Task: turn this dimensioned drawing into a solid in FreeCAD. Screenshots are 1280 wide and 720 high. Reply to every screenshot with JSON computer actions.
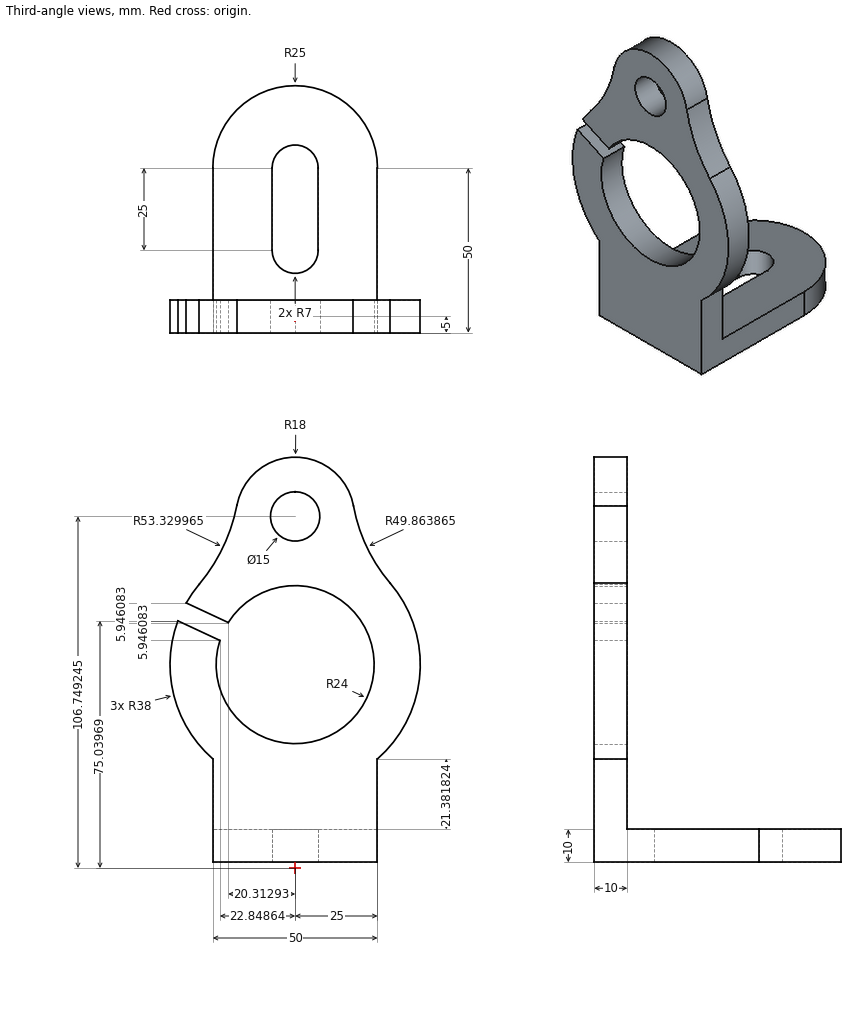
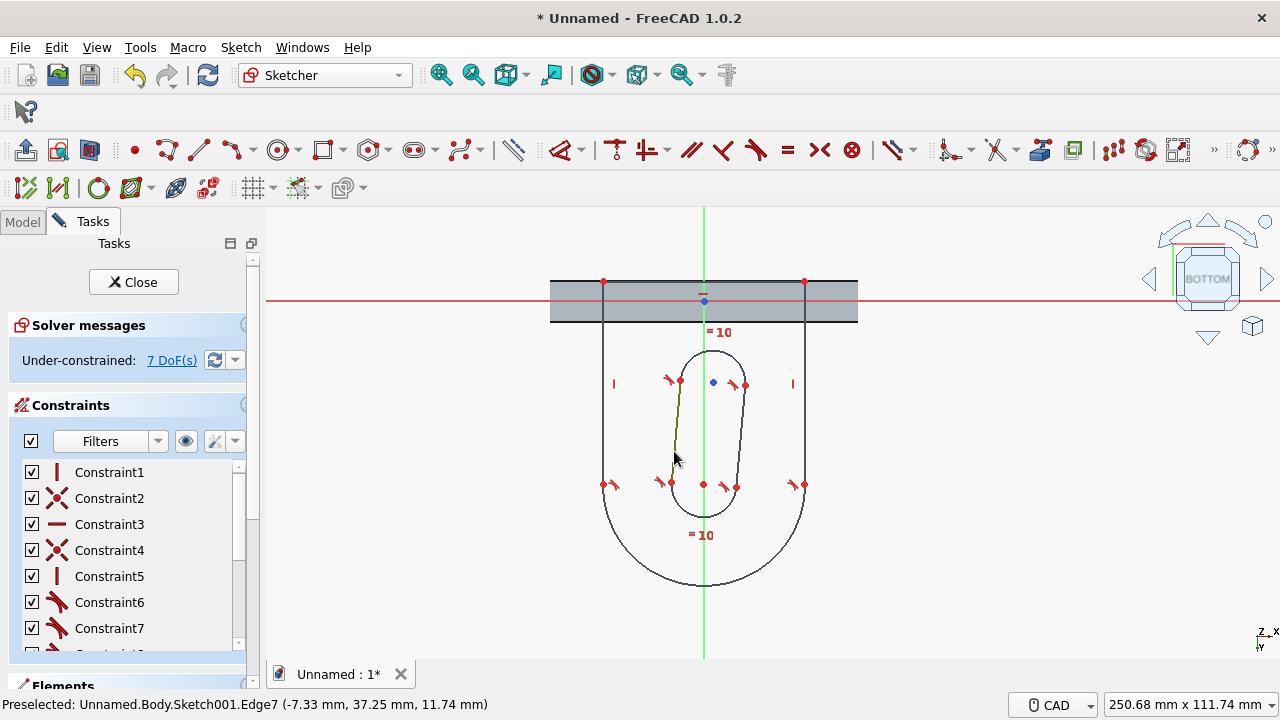
{"action": "key", "text": "v"}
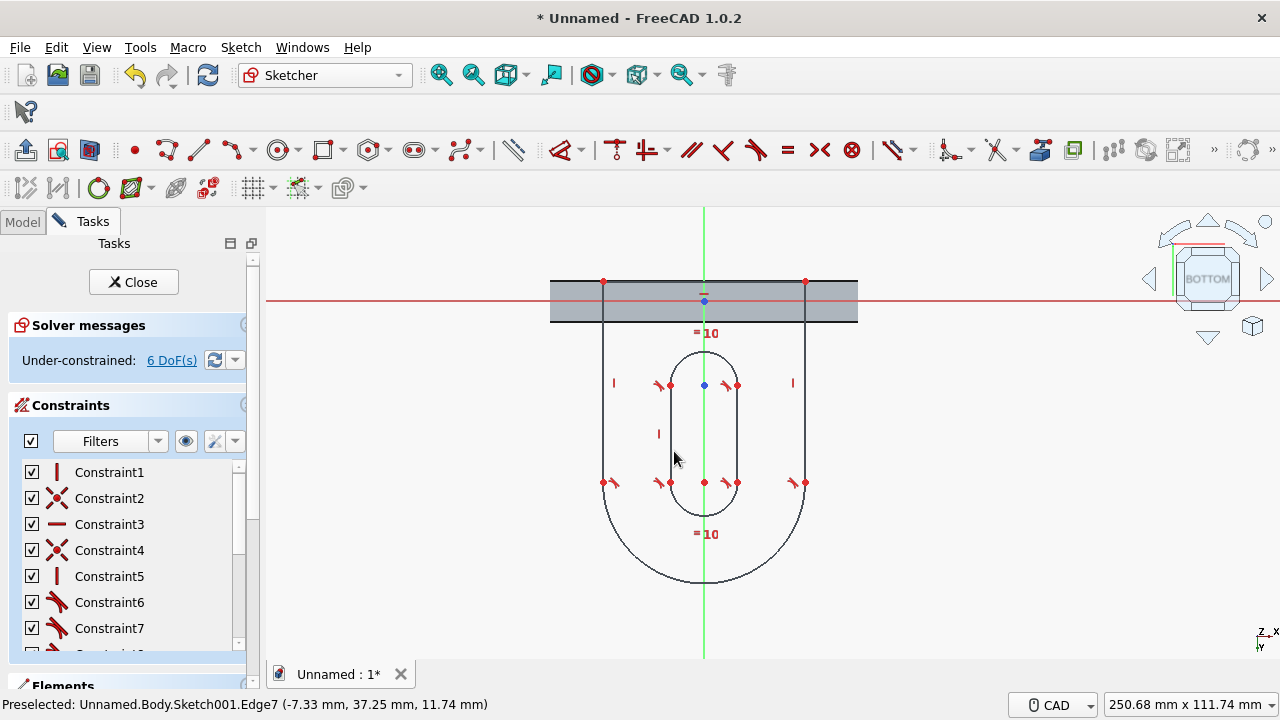
{"action": "left_click", "coordinate": [704, 482]}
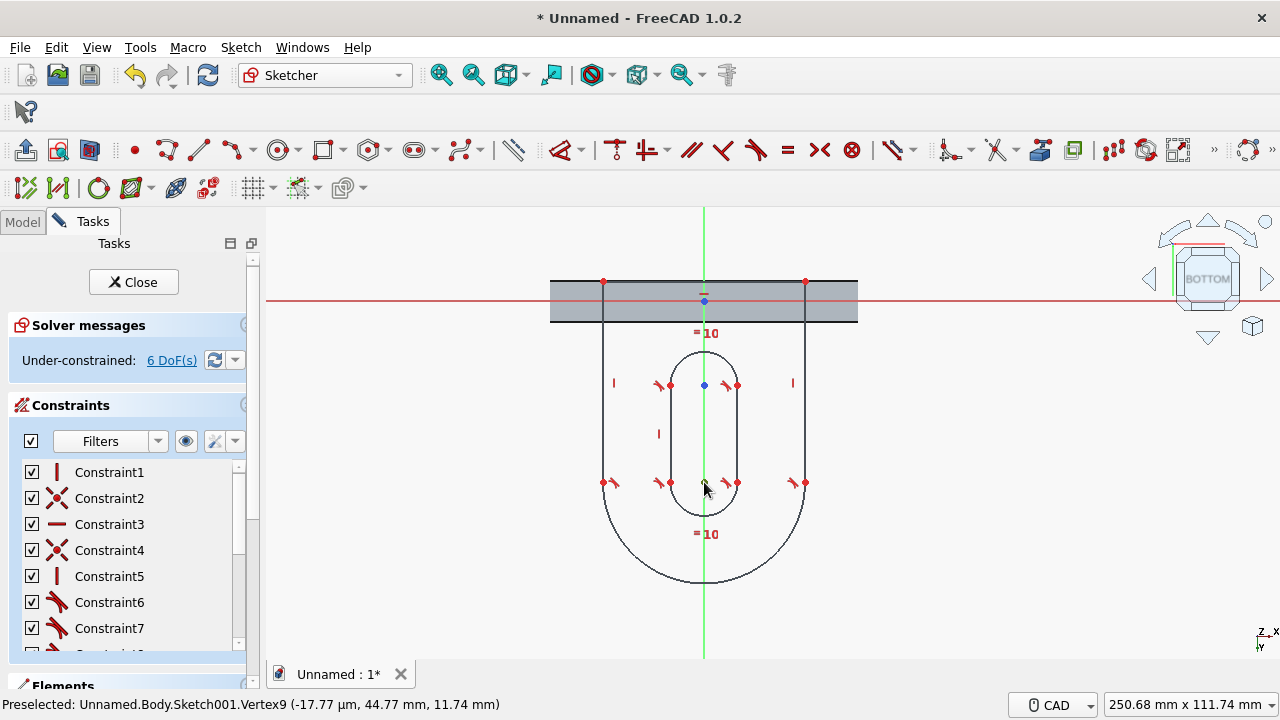
{"action": "left_click", "coordinate": [704, 546]}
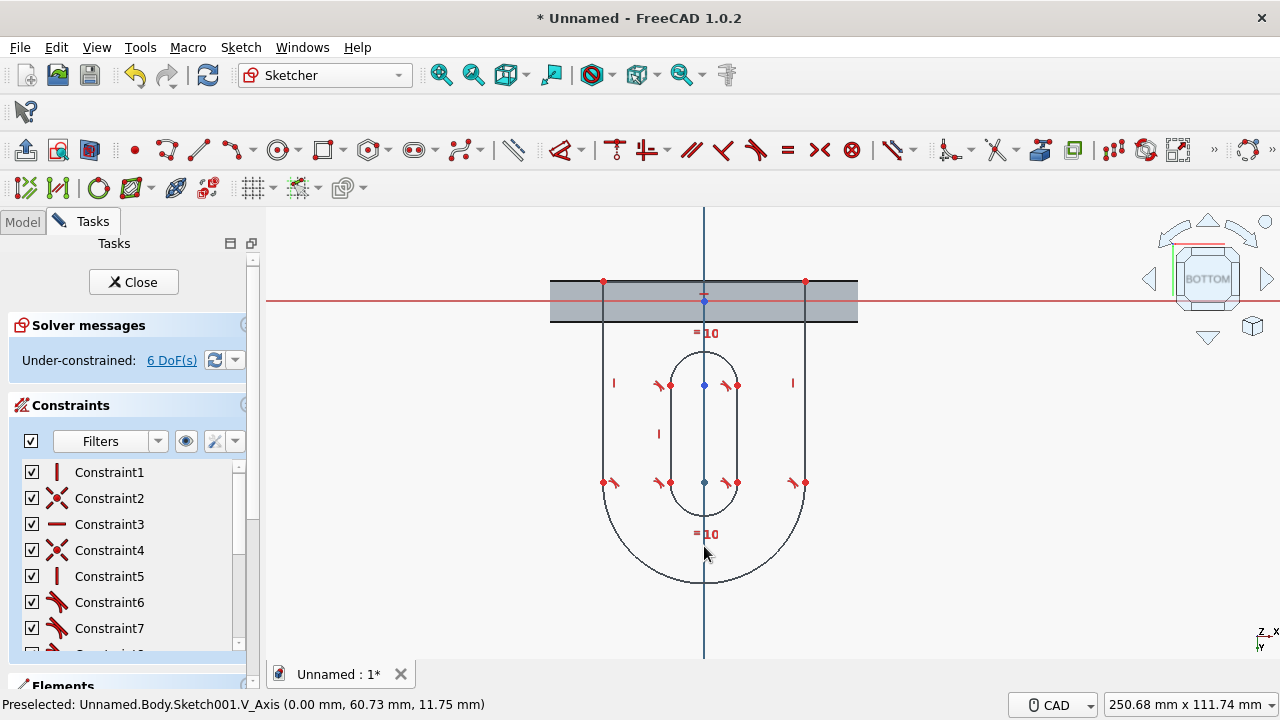
{"action": "left_click", "coordinate": [616, 150]}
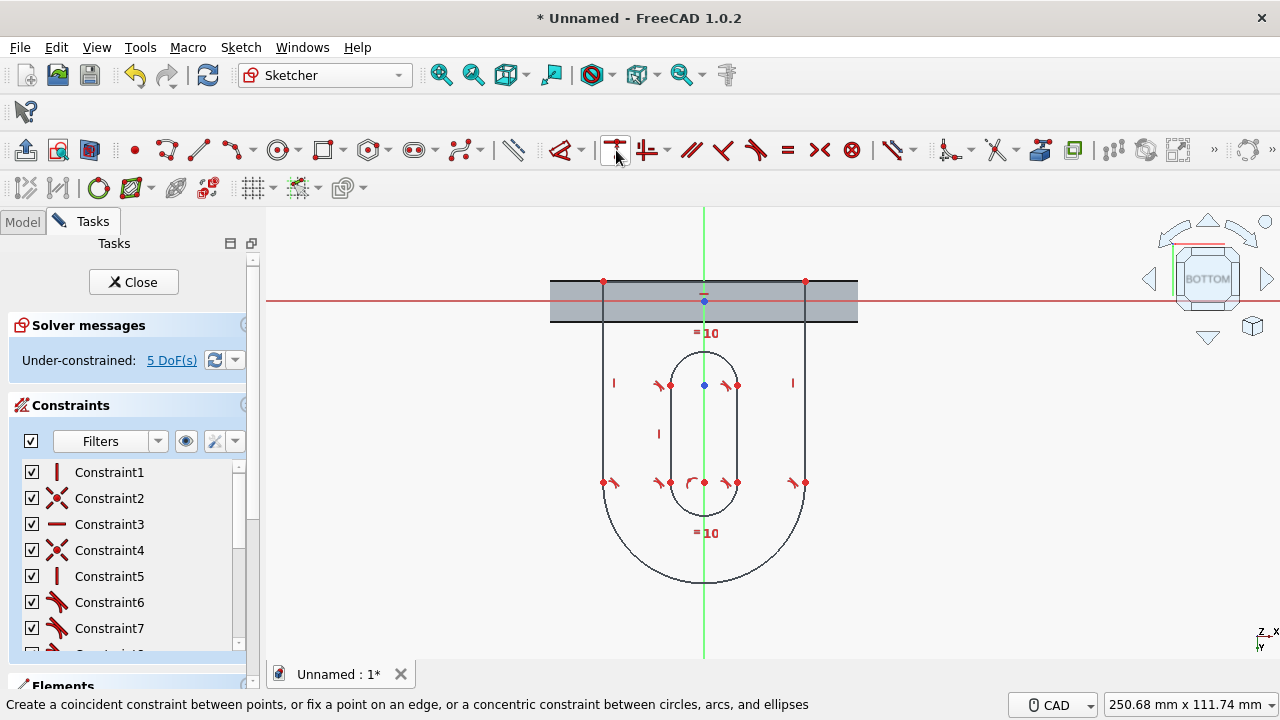
{"action": "left_click", "coordinate": [560, 150]}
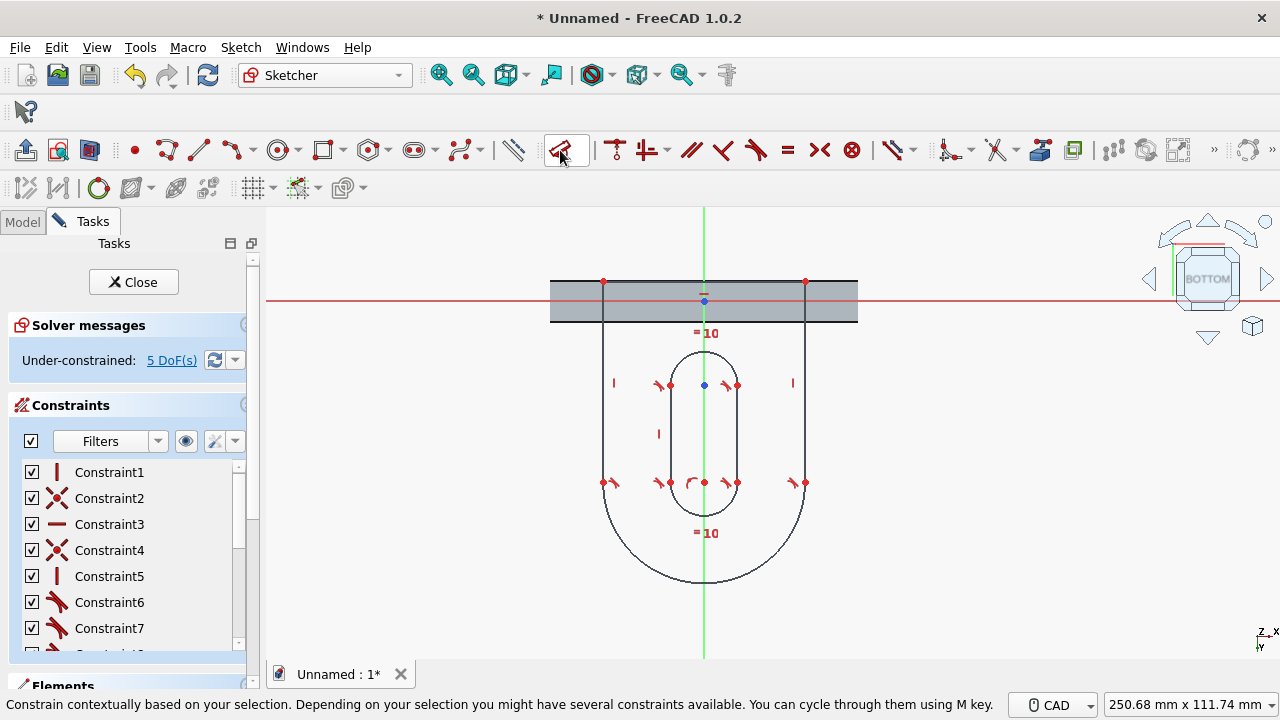
{"action": "left_click", "coordinate": [645, 564]}
{"action": "left_click", "coordinate": [626, 590]}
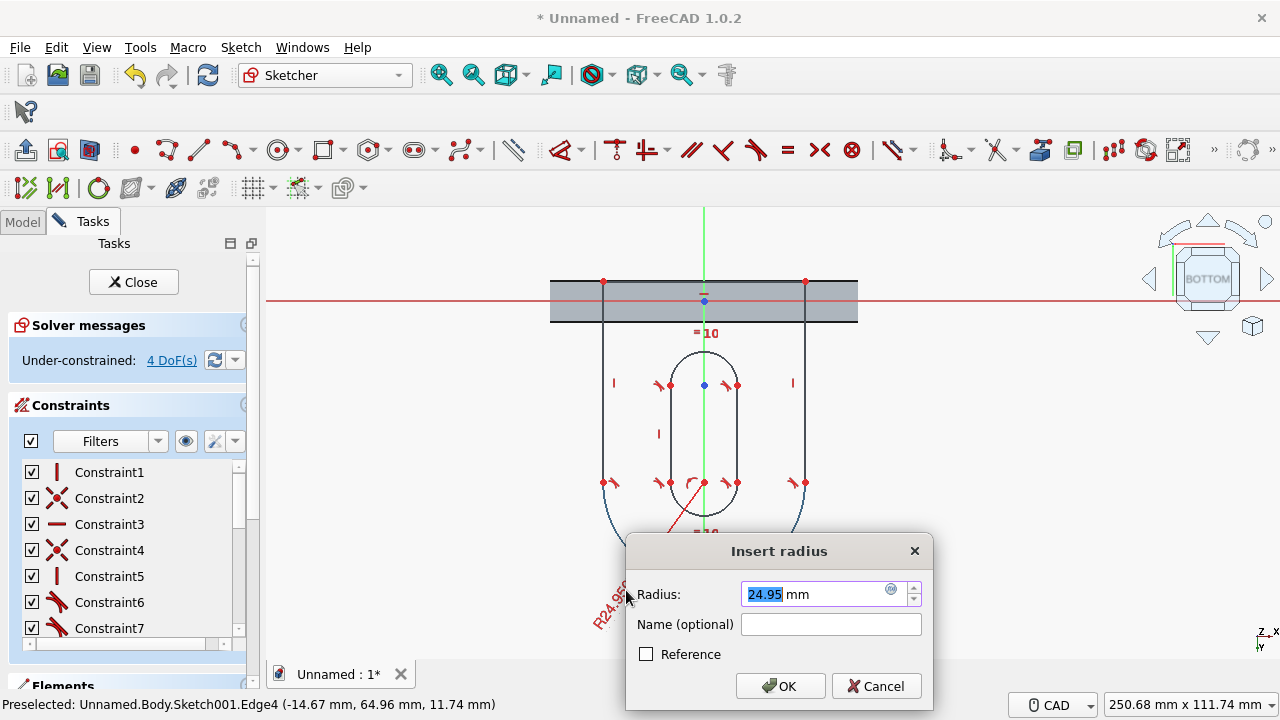
{"action": "type", "text": "25"}
{"action": "key", "text": "Return"}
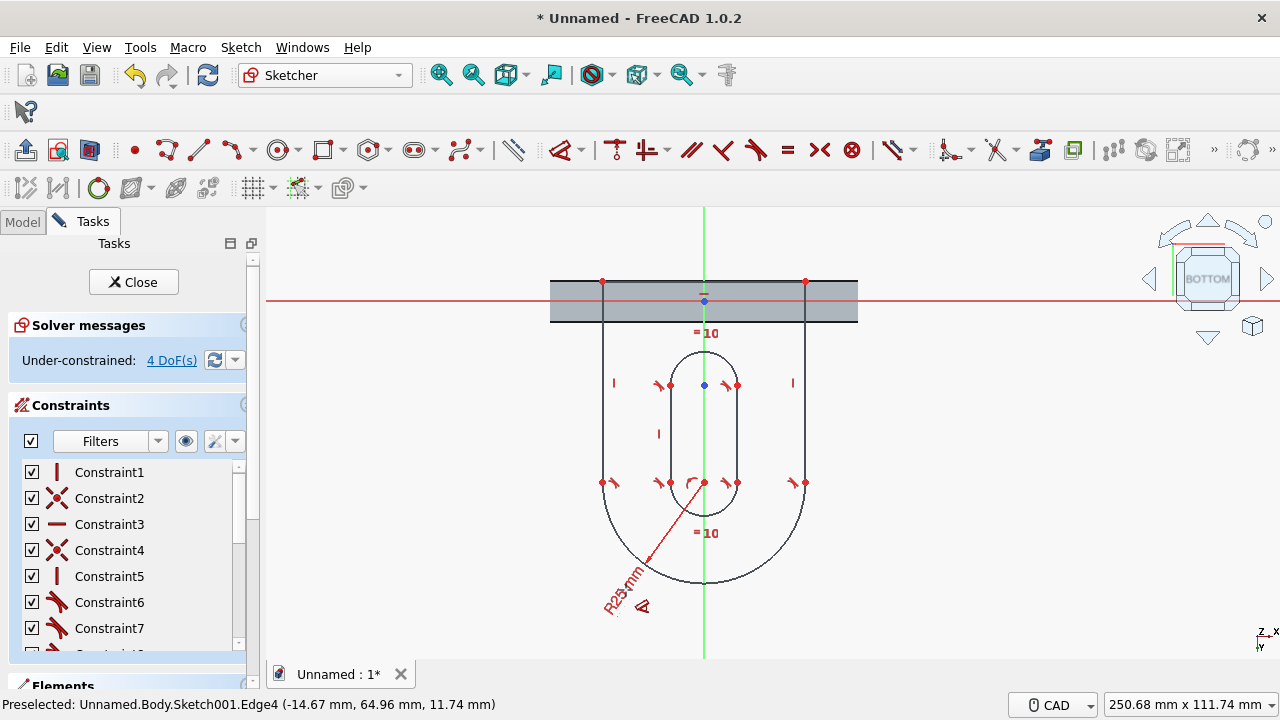
{"action": "scroll", "coordinate": [684, 509], "scroll_direction": "up", "scroll_amount": 2}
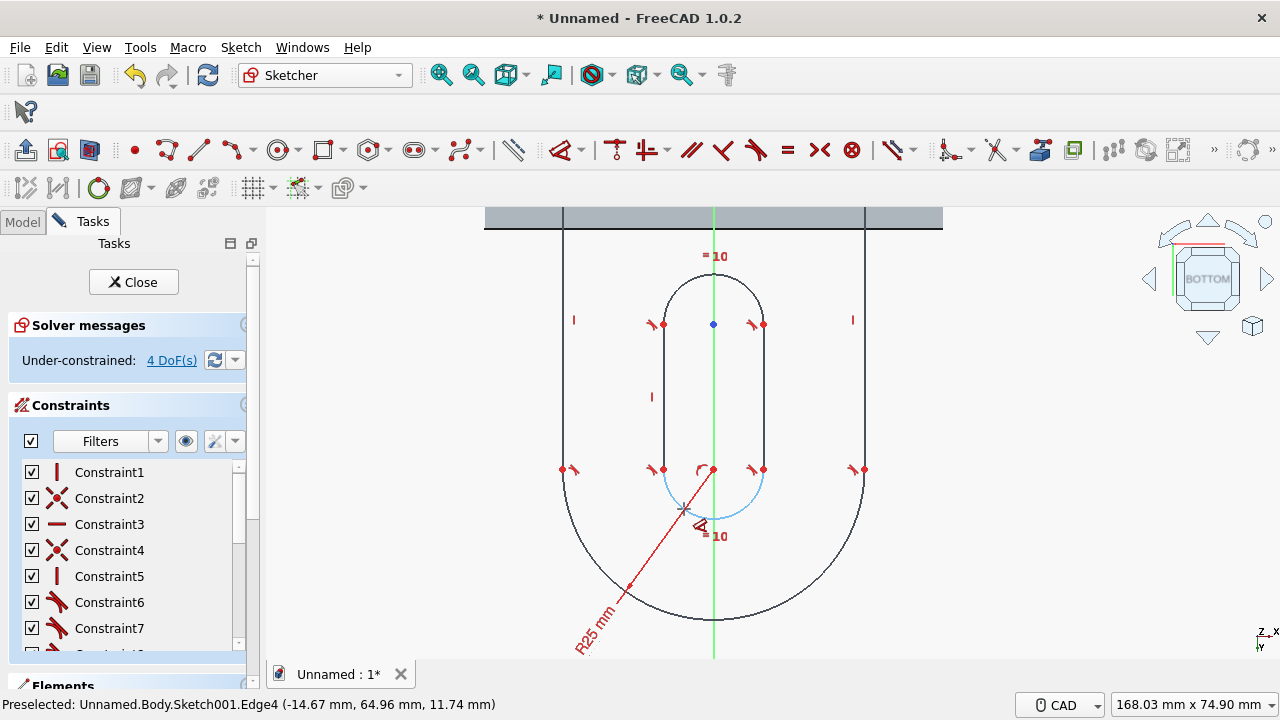
{"action": "left_click", "coordinate": [684, 509]}
{"action": "left_click", "coordinate": [665, 535]}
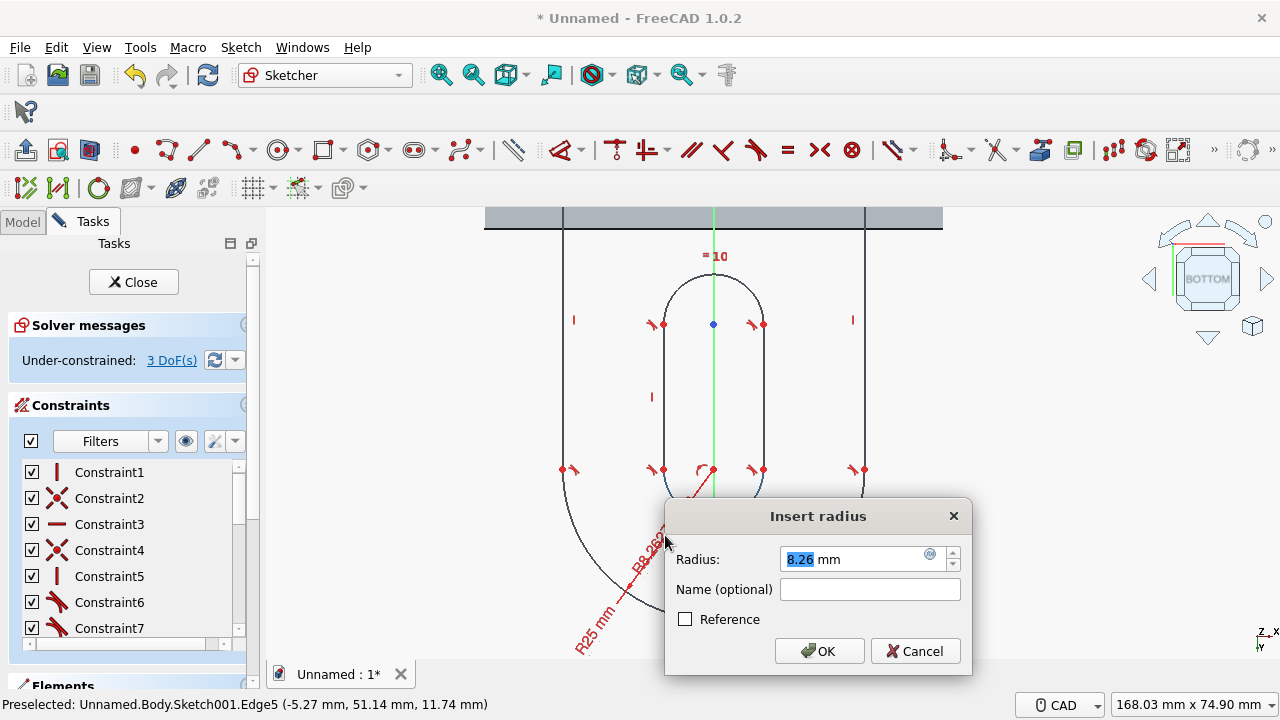
{"action": "type", "text": "7"}
{"action": "key", "text": "Return"}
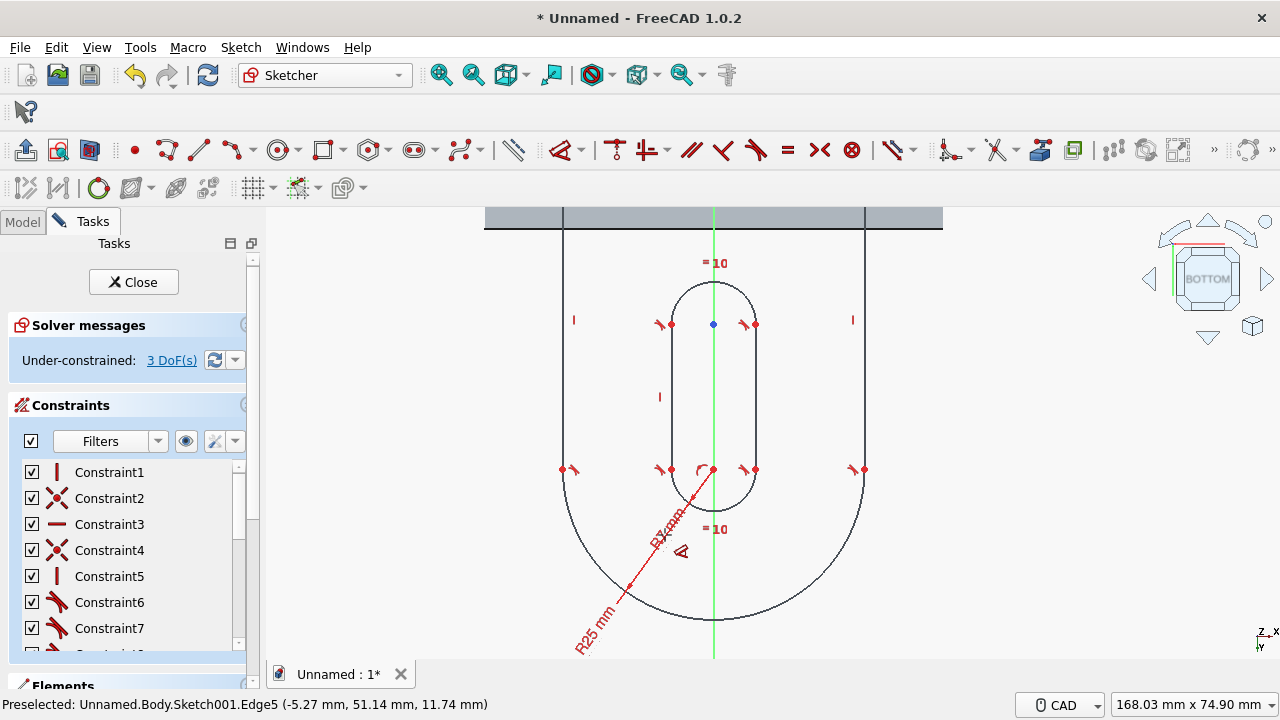
{"action": "left_click", "coordinate": [865, 379]}
{"action": "left_click", "coordinate": [899, 352]}